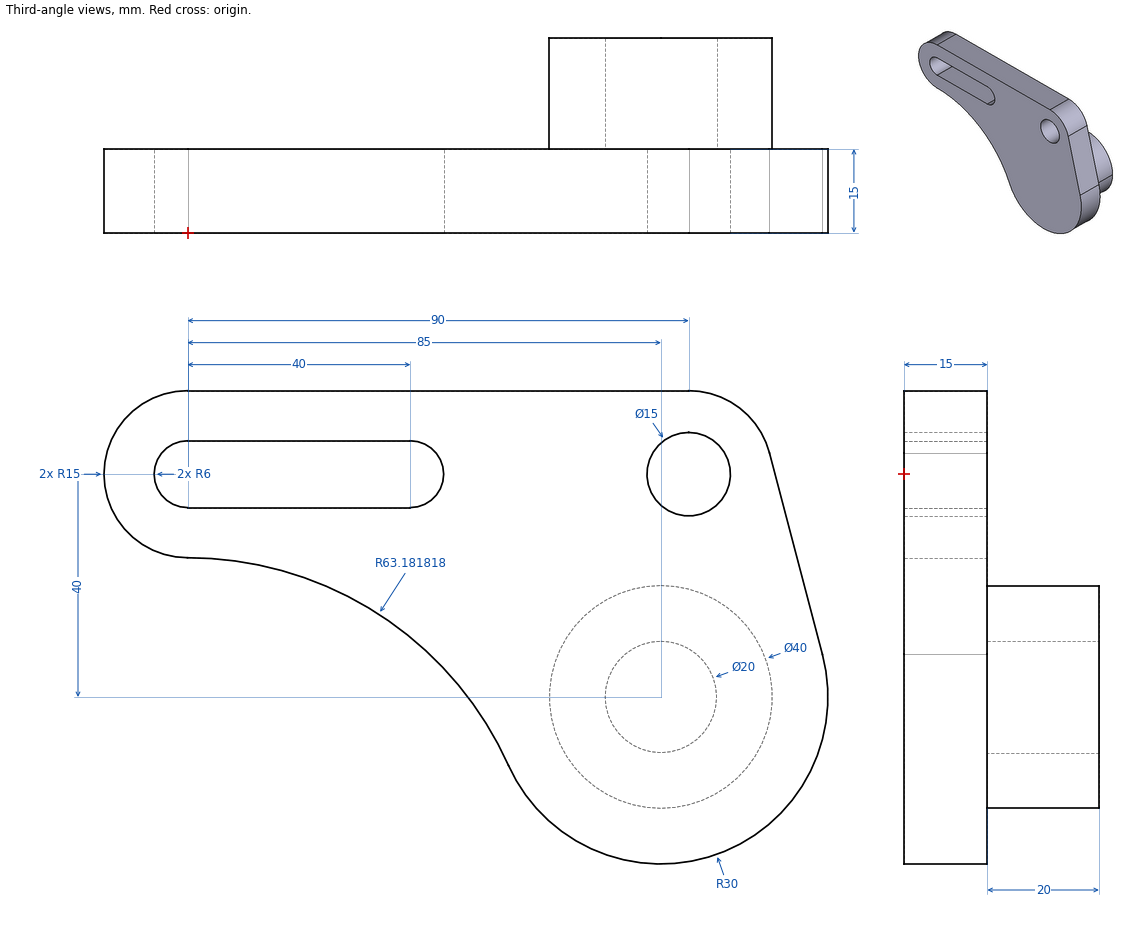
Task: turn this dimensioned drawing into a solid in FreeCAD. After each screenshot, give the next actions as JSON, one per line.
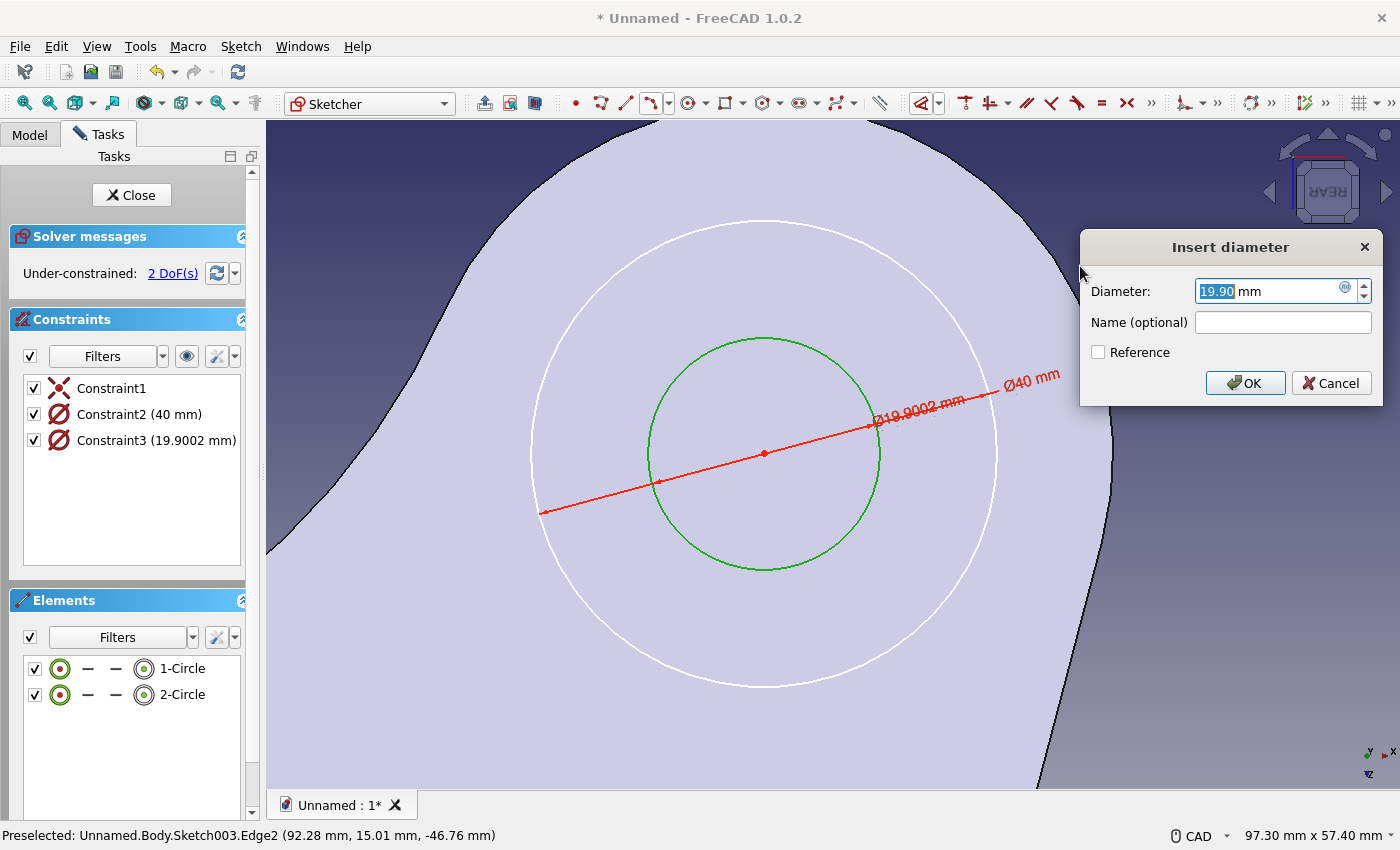
{"action": "type", "text": "20"}
{"action": "key", "text": "Return"}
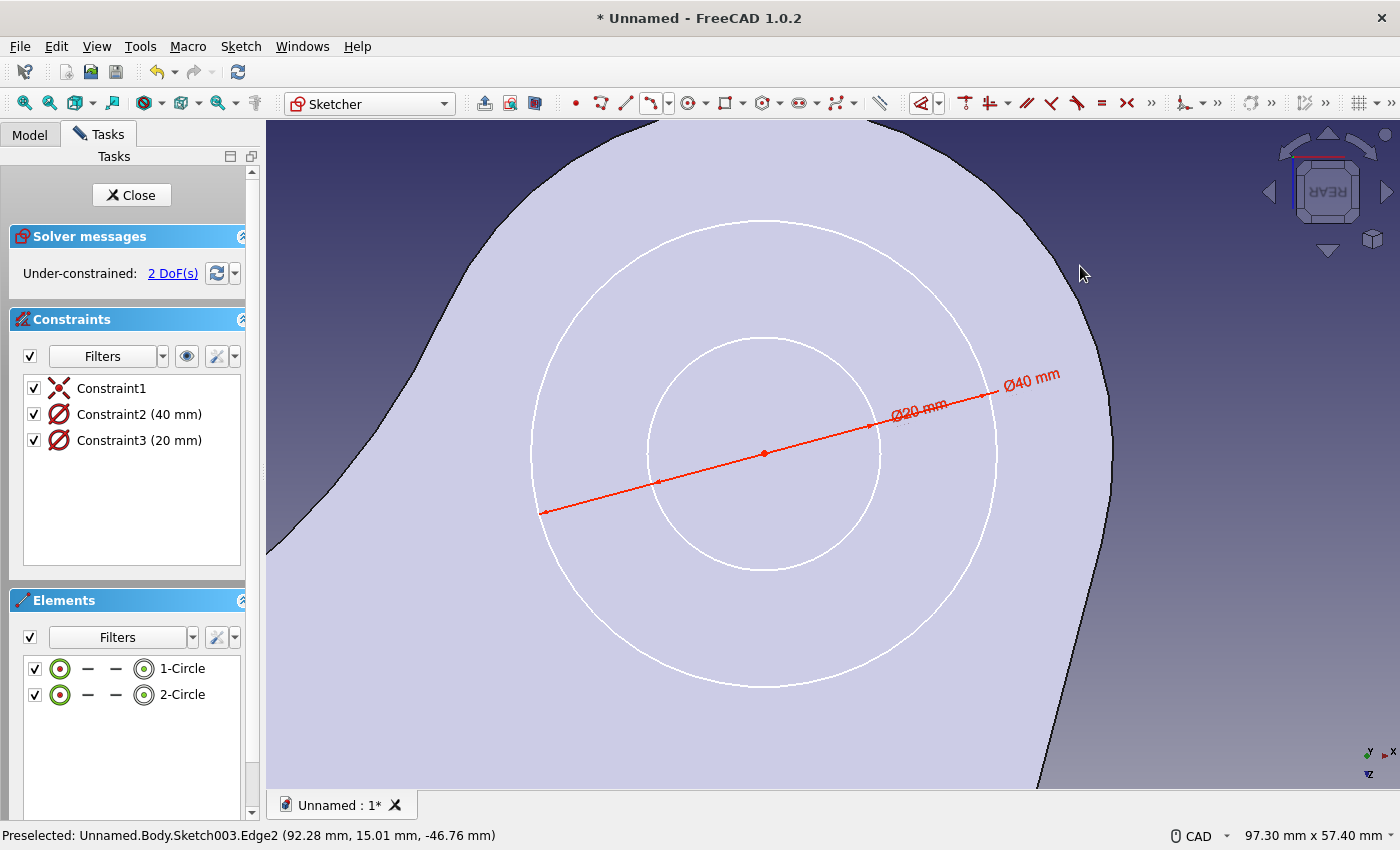
{"action": "left_click", "coordinate": [764, 454]}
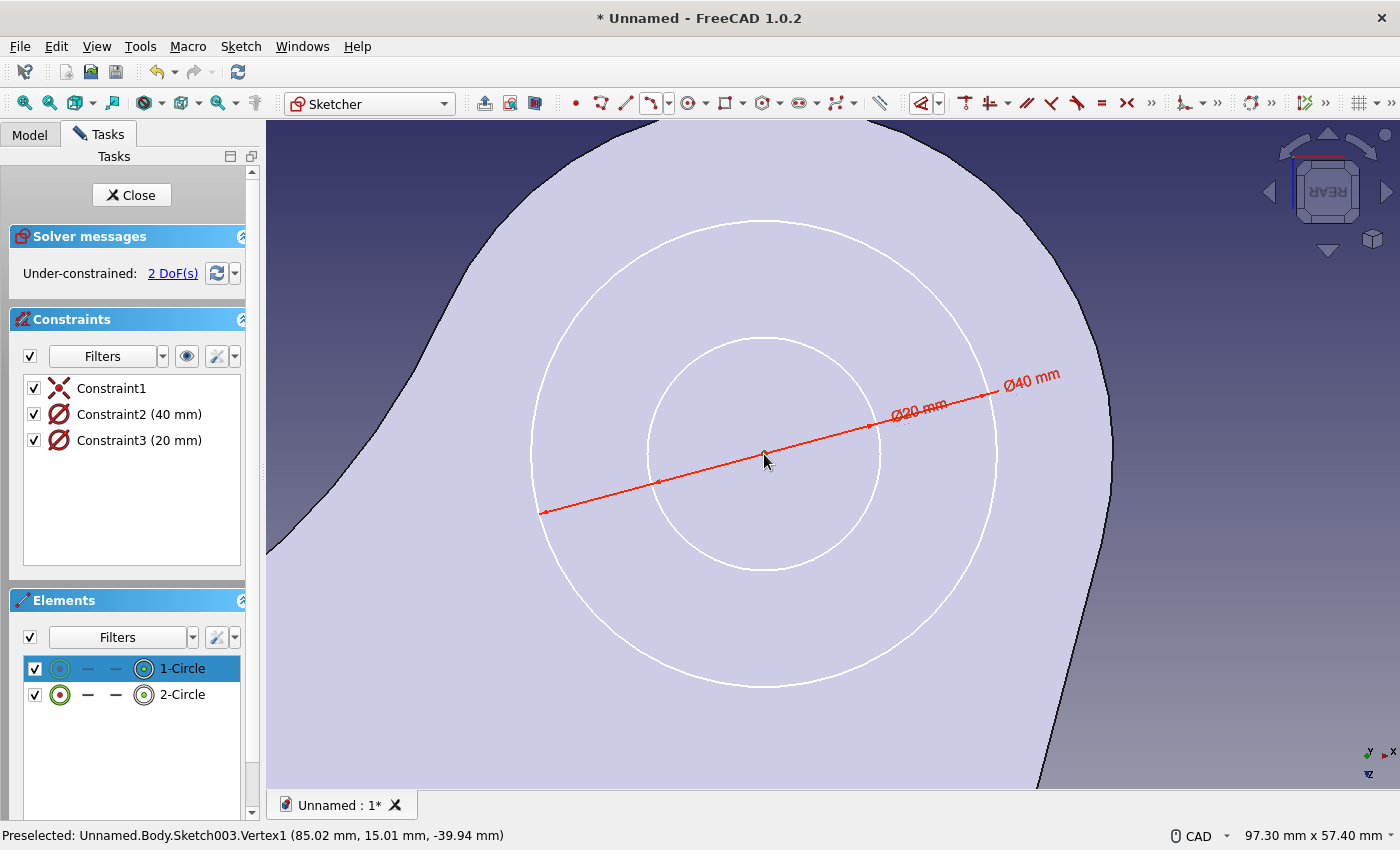
{"action": "left_click", "coordinate": [938, 104]}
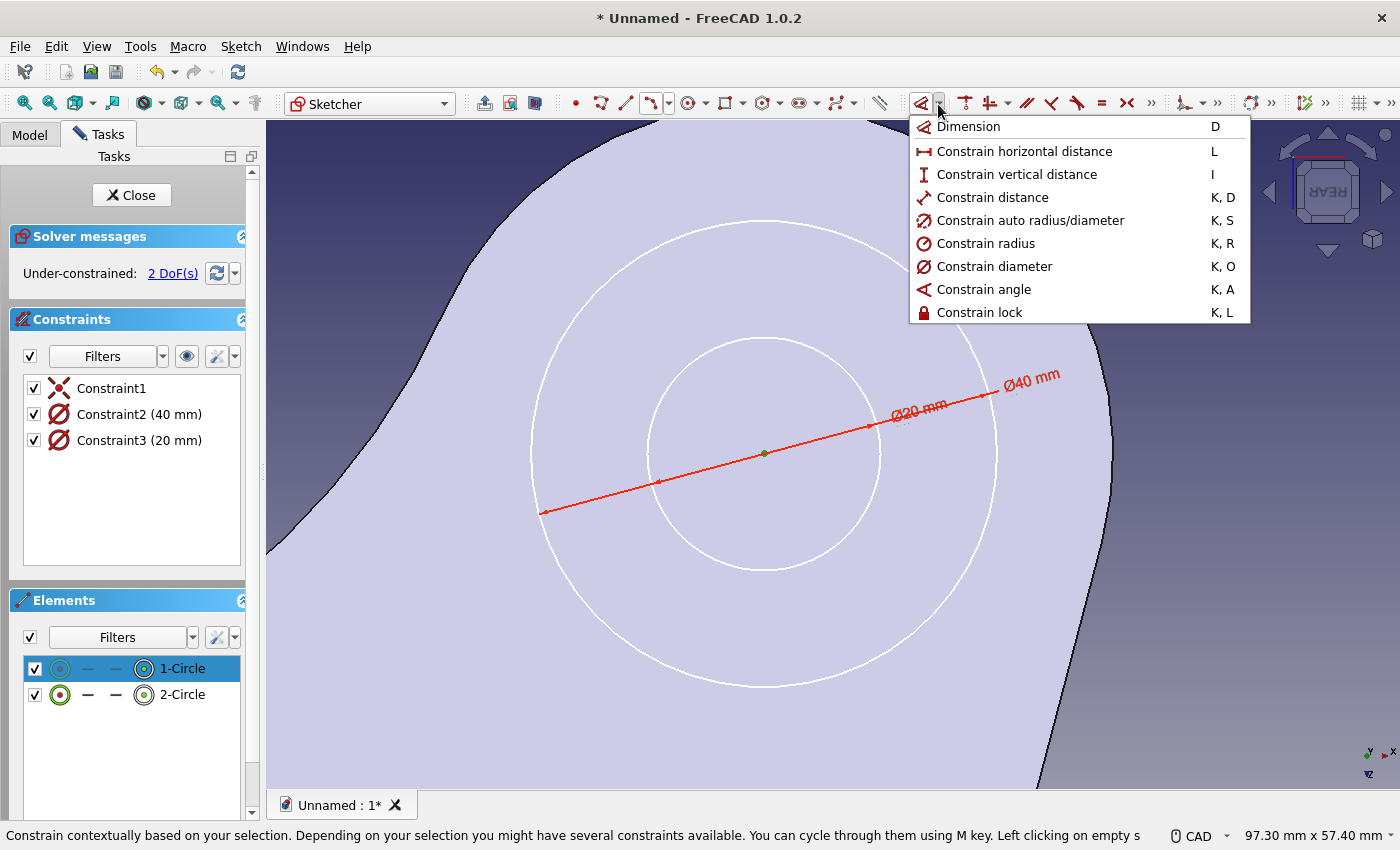
{"action": "left_click", "coordinate": [1080, 152]}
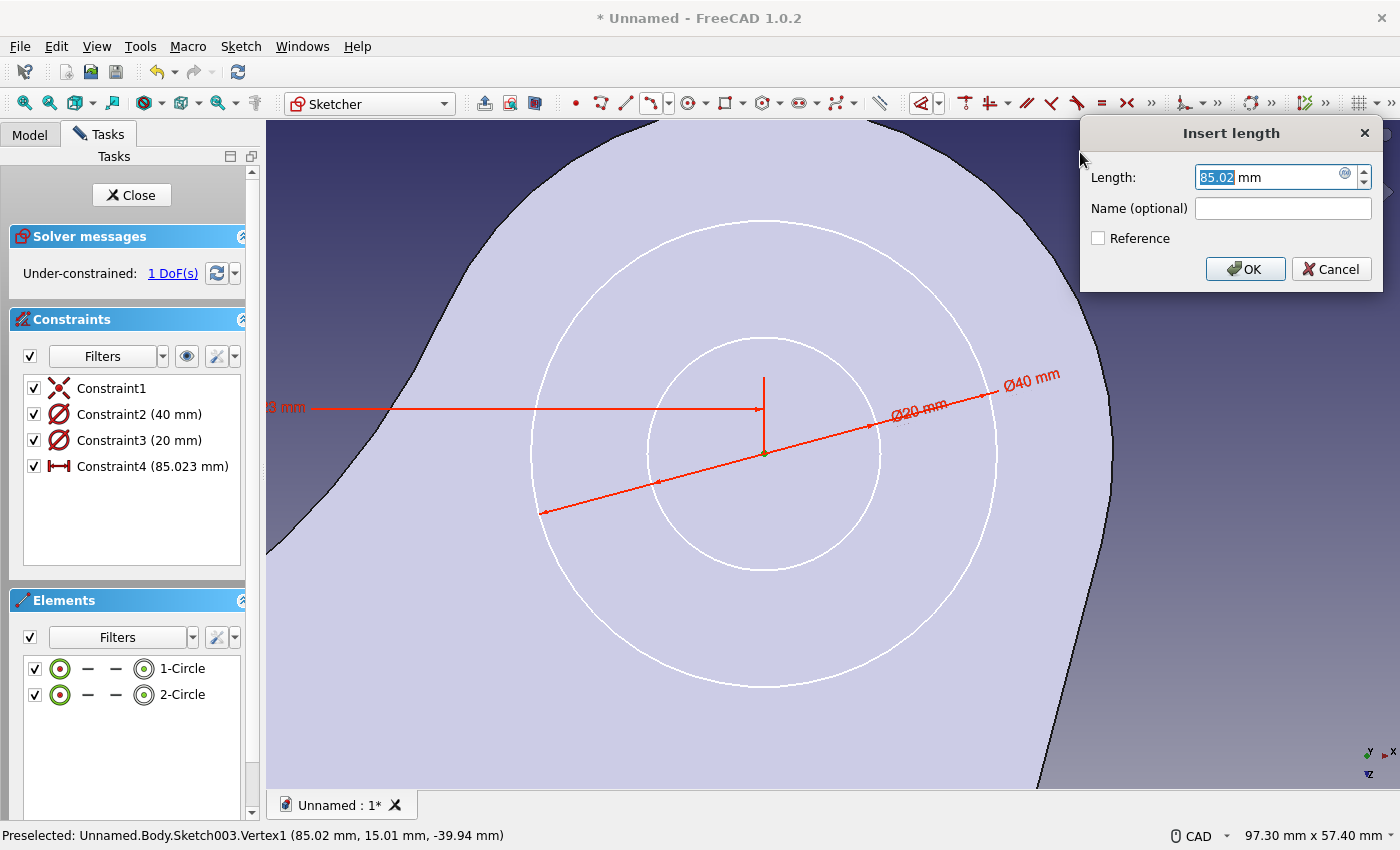
{"action": "type", "text": "85"}
{"action": "key", "text": "Return"}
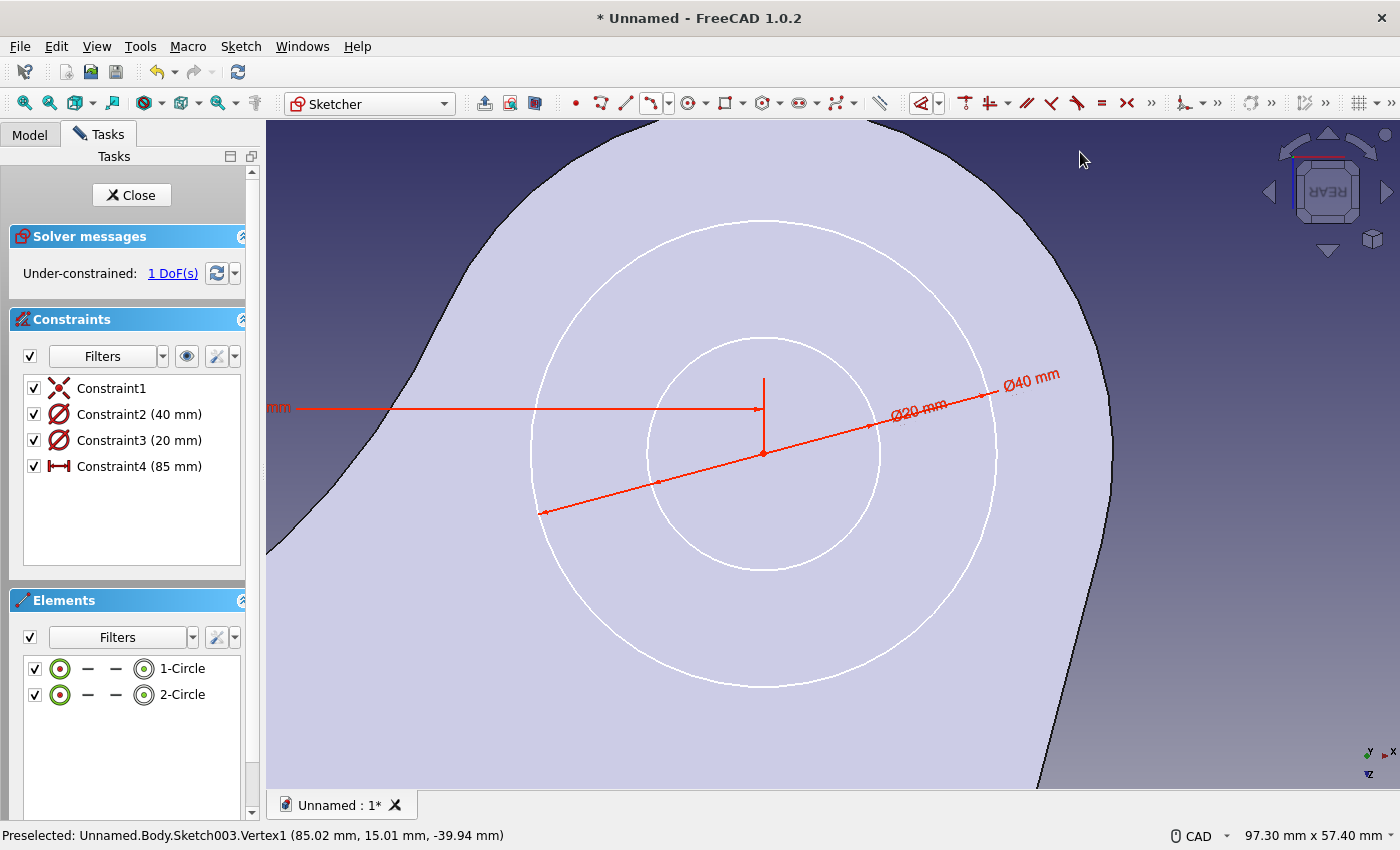
{"action": "left_click", "coordinate": [764, 454]}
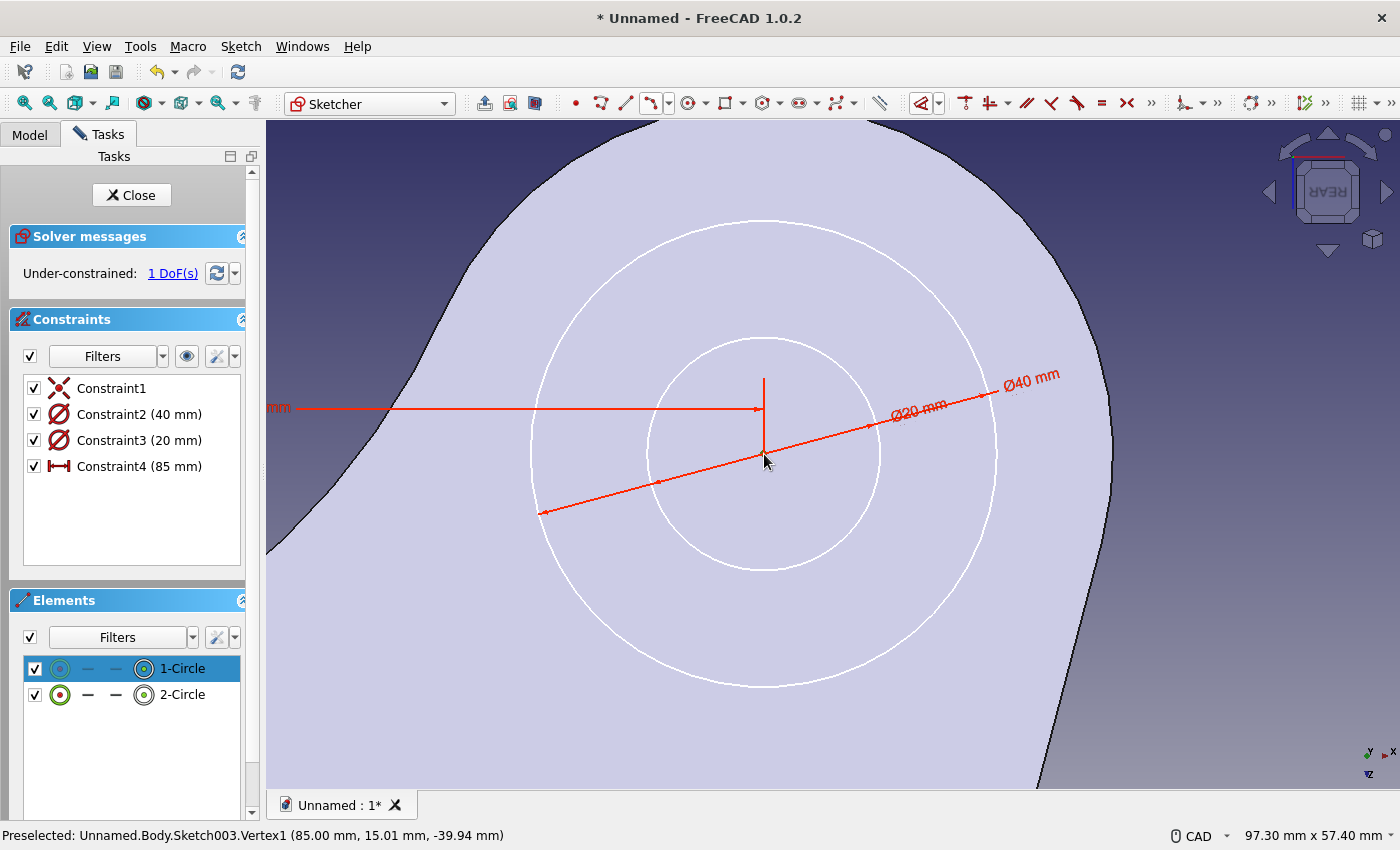
{"action": "key", "text": "i"}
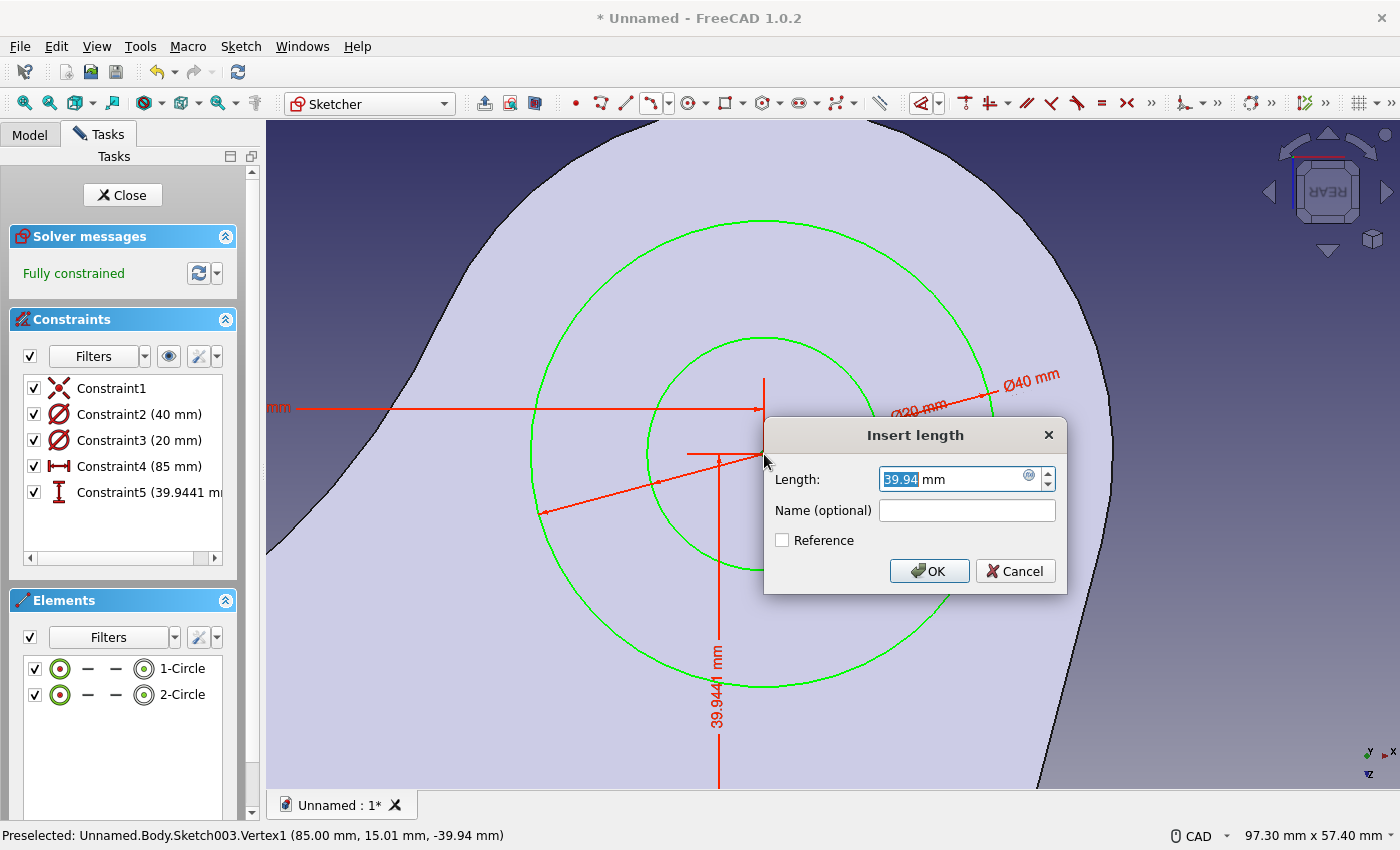
{"action": "type", "text": "40"}
{"action": "key", "text": "Return"}